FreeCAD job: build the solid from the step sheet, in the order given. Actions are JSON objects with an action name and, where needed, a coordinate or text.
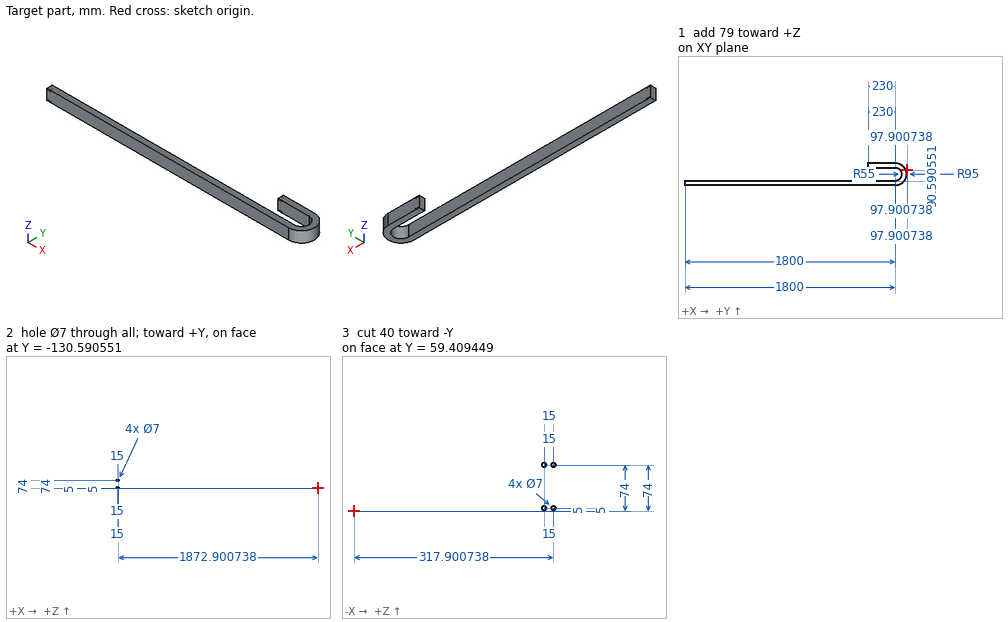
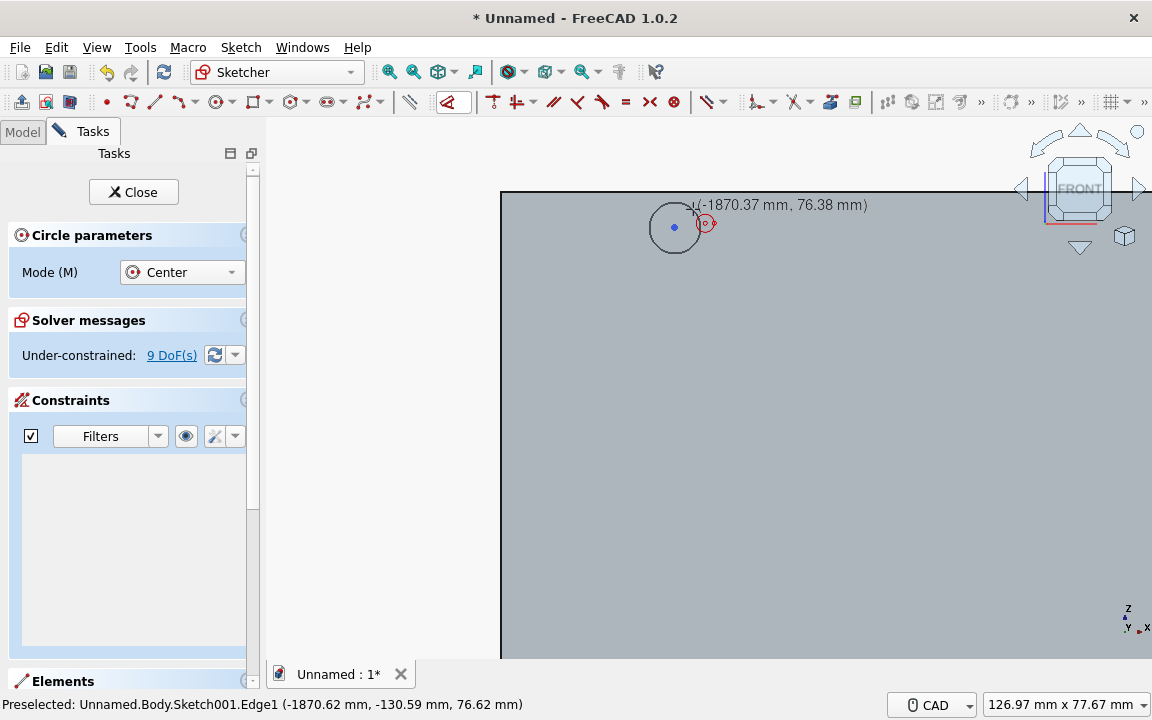
{"action": "left_click", "coordinate": [571, 227]}
{"action": "left_click", "coordinate": [588, 209]}
{"action": "key", "text": "Escape"}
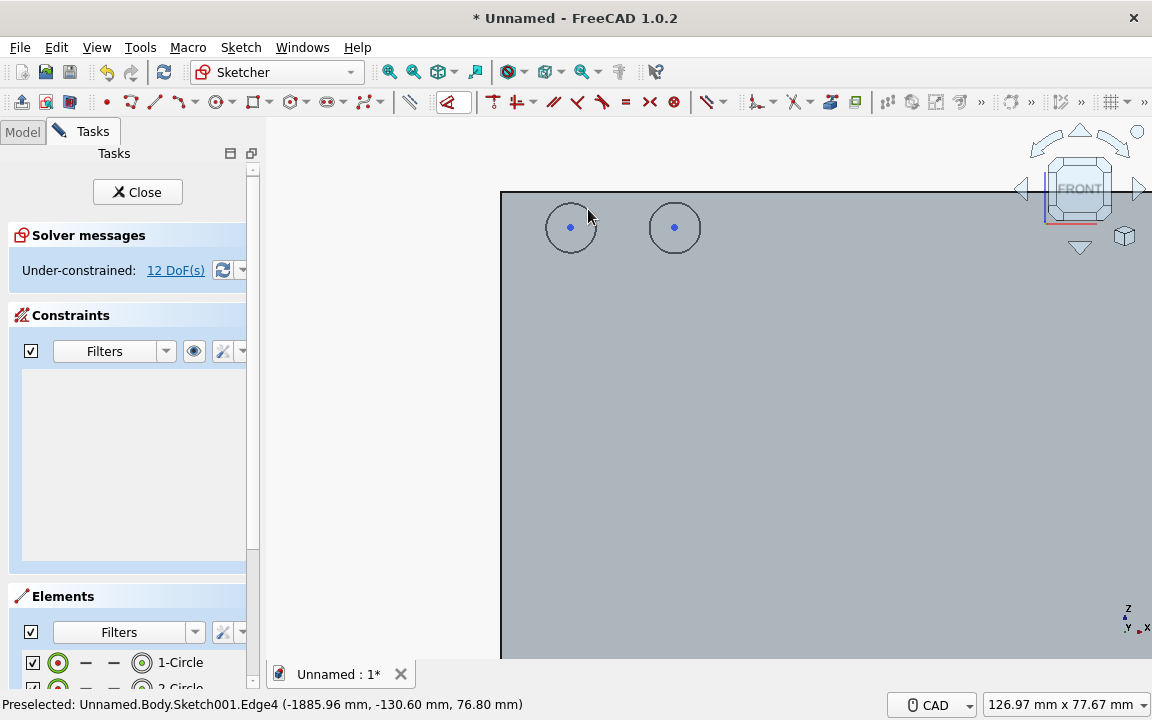
{"action": "scroll", "coordinate": [676, 227], "scroll_direction": "down", "scroll_amount": 2}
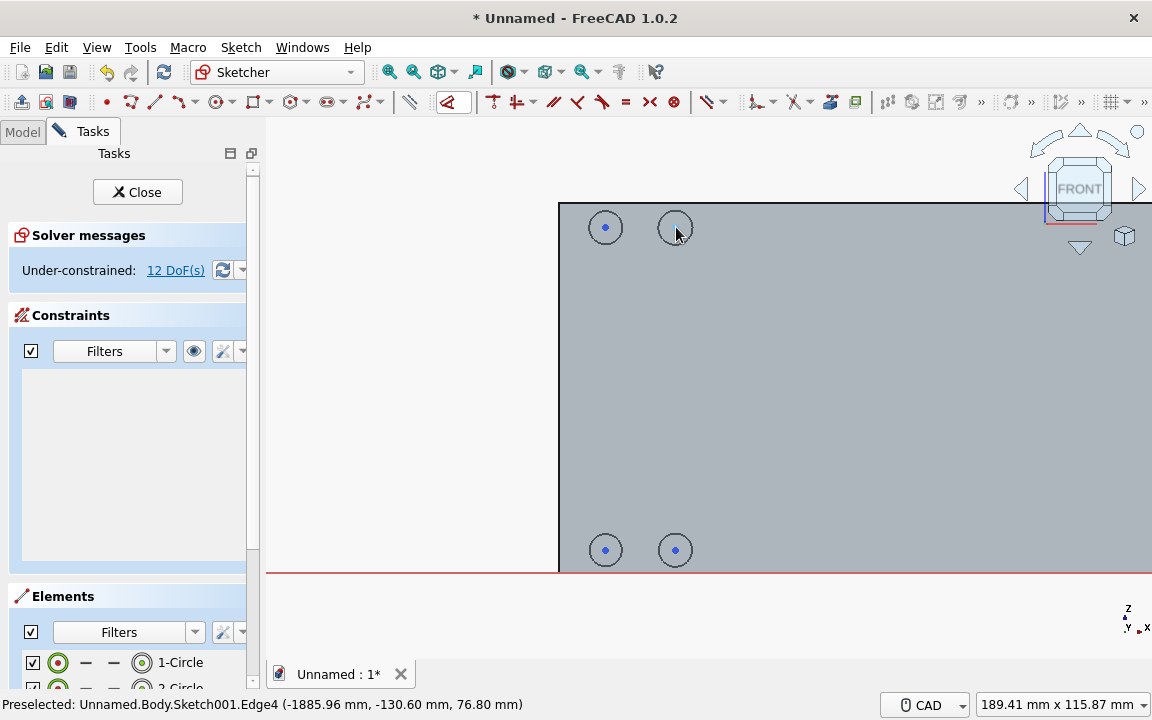
{"action": "left_click", "coordinate": [687, 538]}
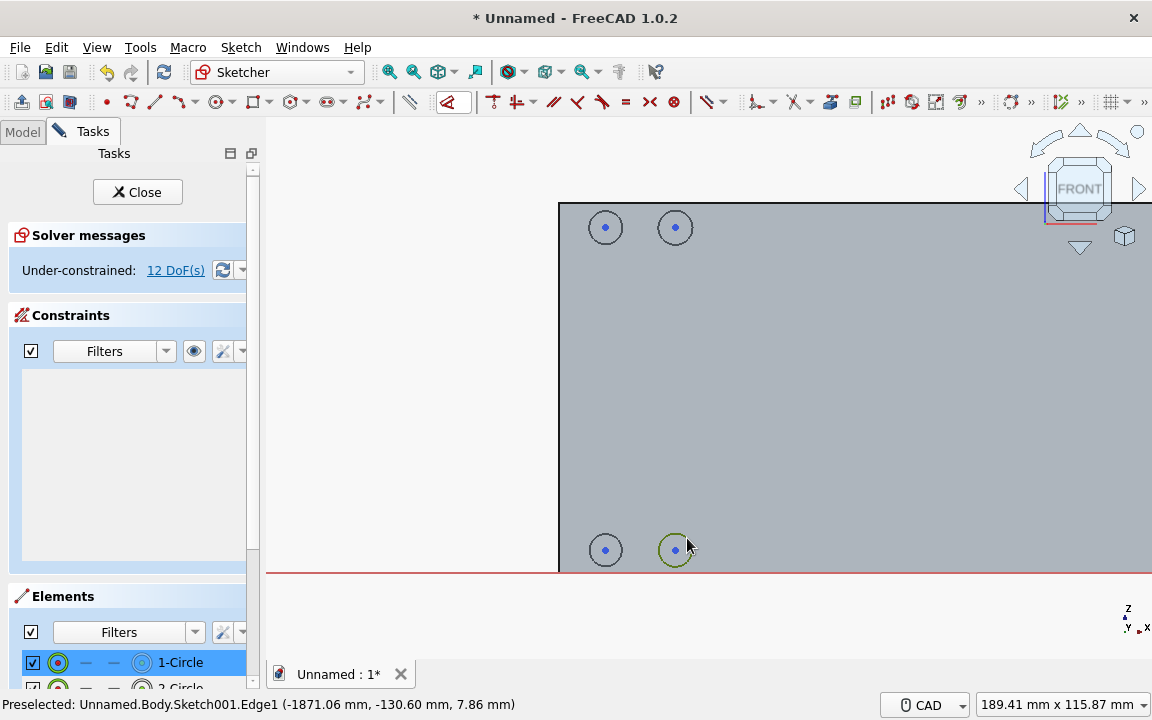
{"action": "left_click", "coordinate": [617, 539]}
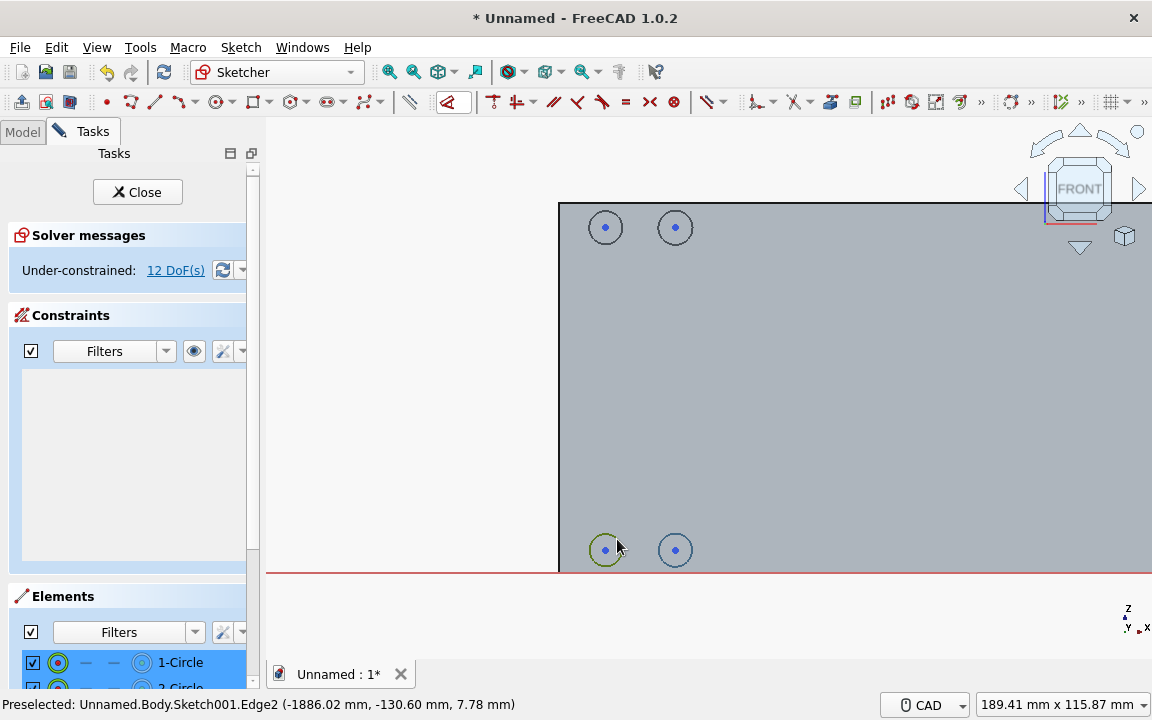
{"action": "left_click", "coordinate": [688, 216]}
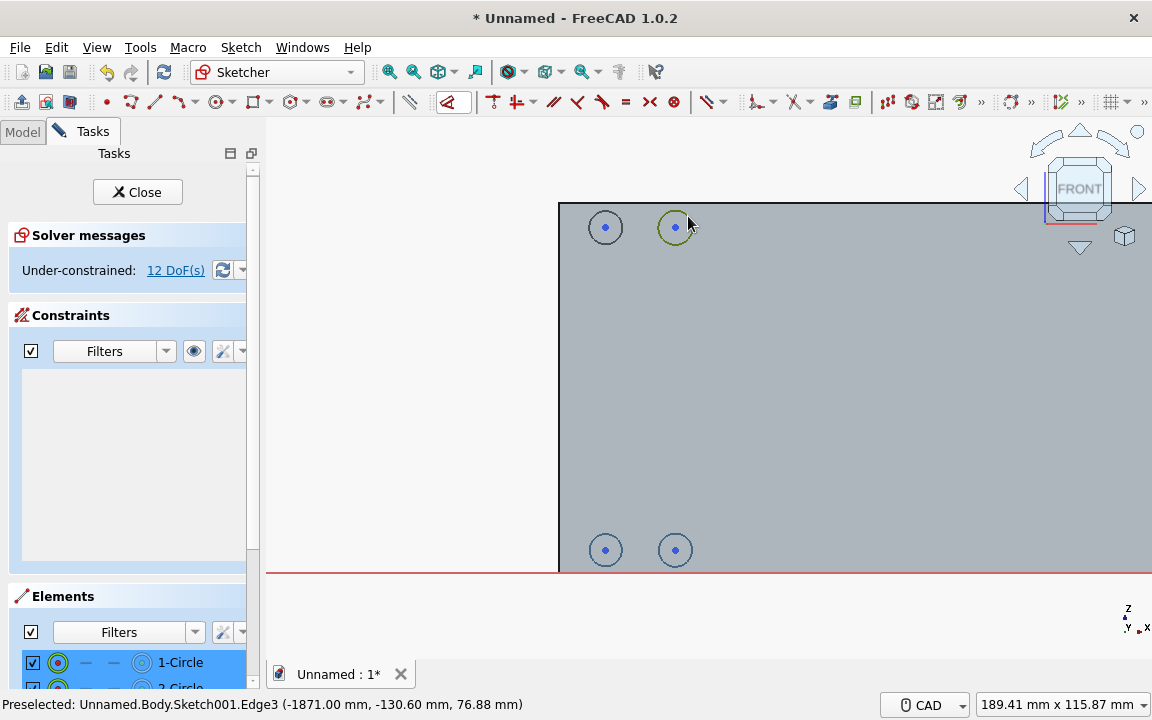
{"action": "left_click", "coordinate": [617, 216]}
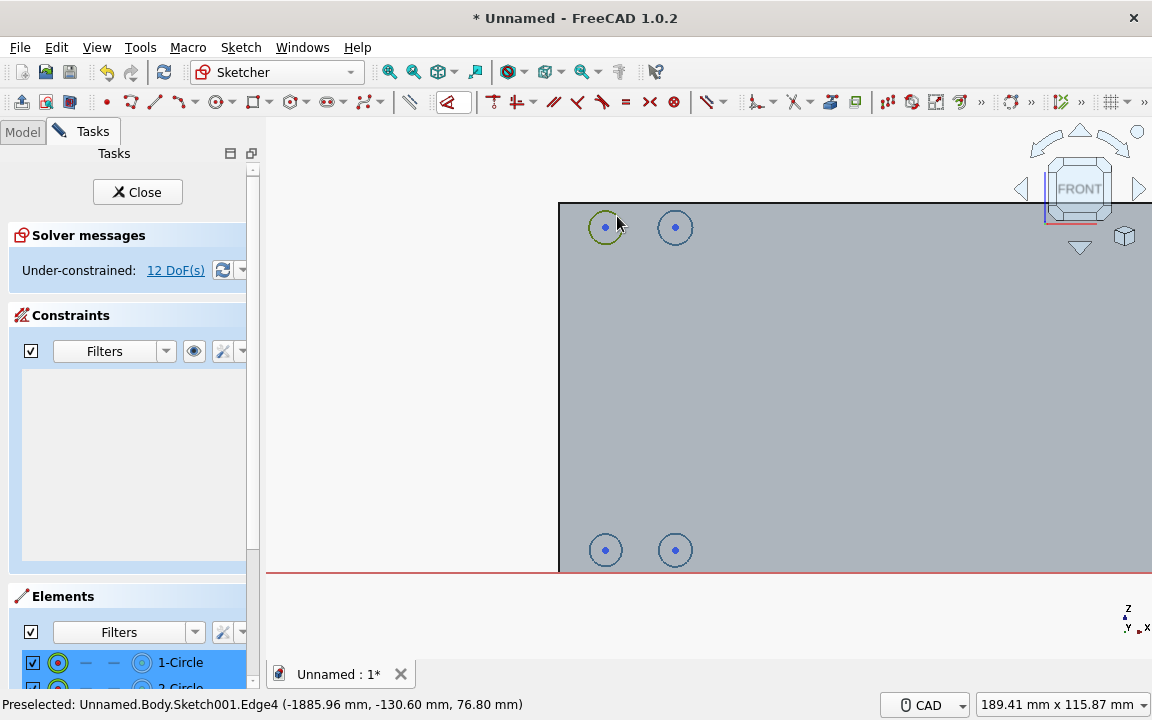
{"action": "left_click", "coordinate": [626, 102]}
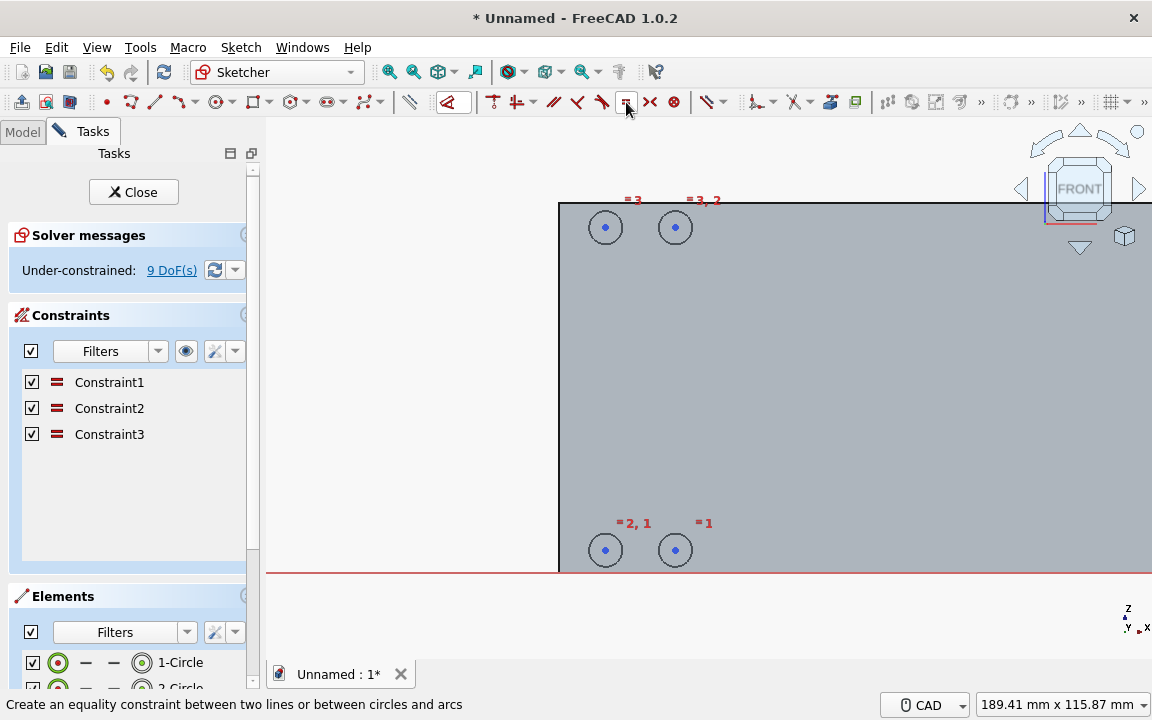
{"action": "key", "text": "d"}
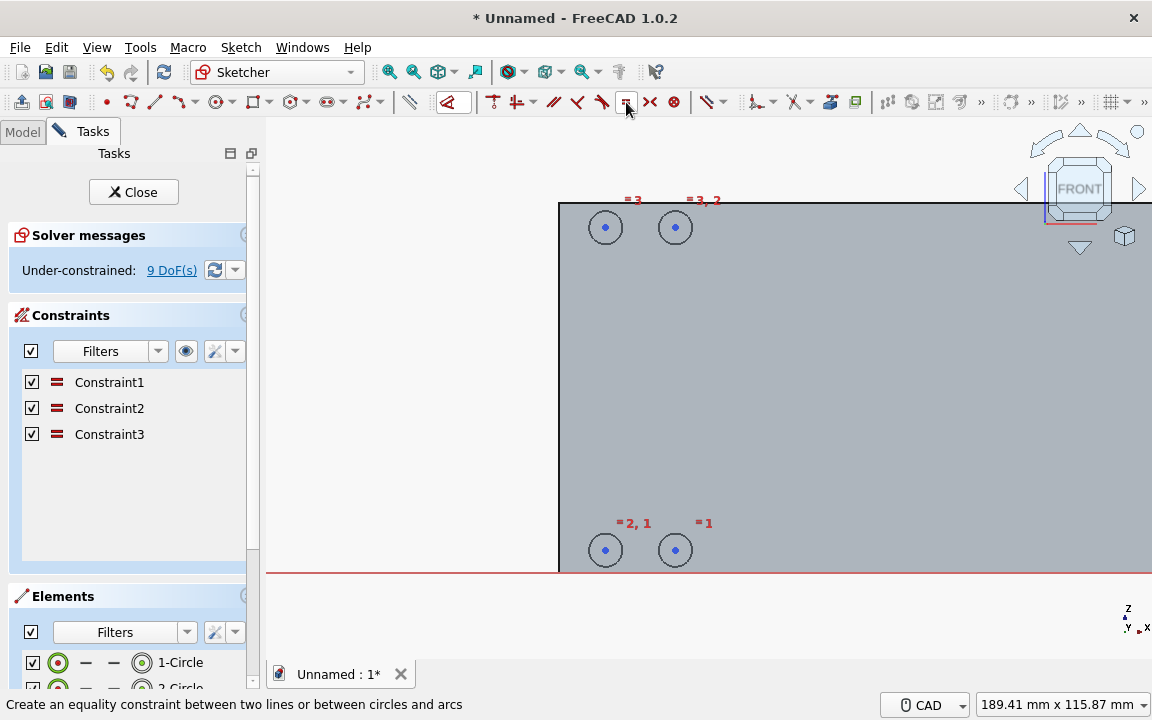
{"action": "left_click", "coordinate": [687, 538]}
{"action": "left_click", "coordinate": [709, 515]}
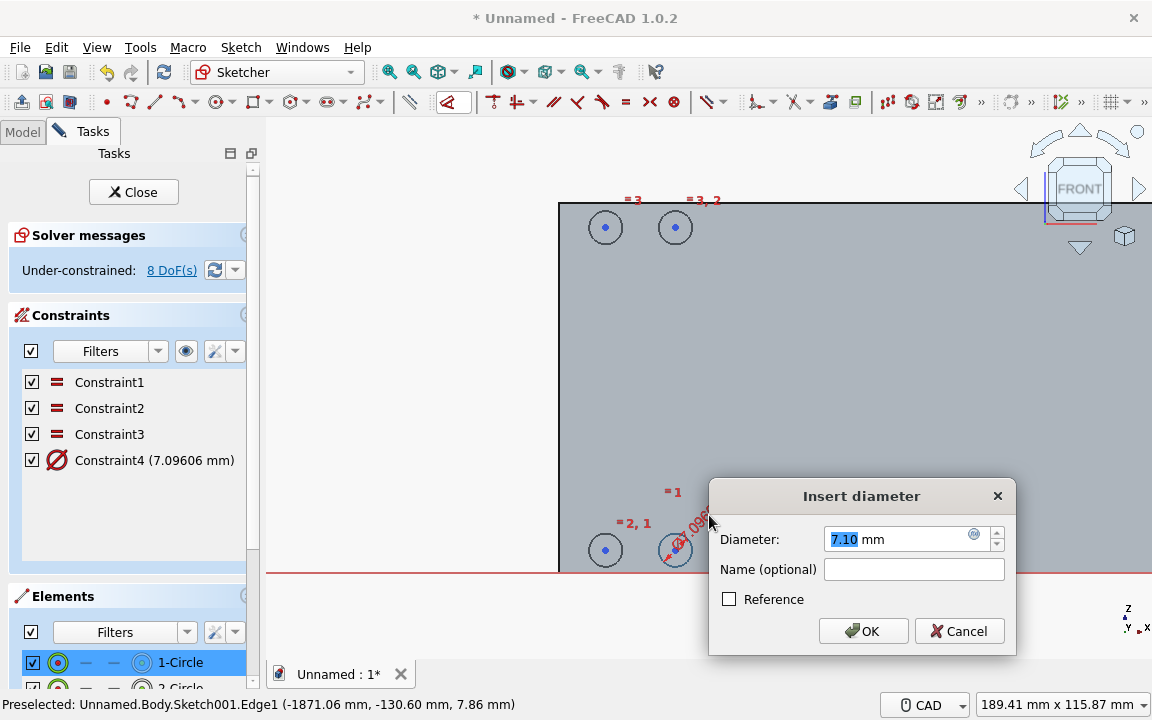
{"action": "type", "text": "7"}
{"action": "key", "text": "Return"}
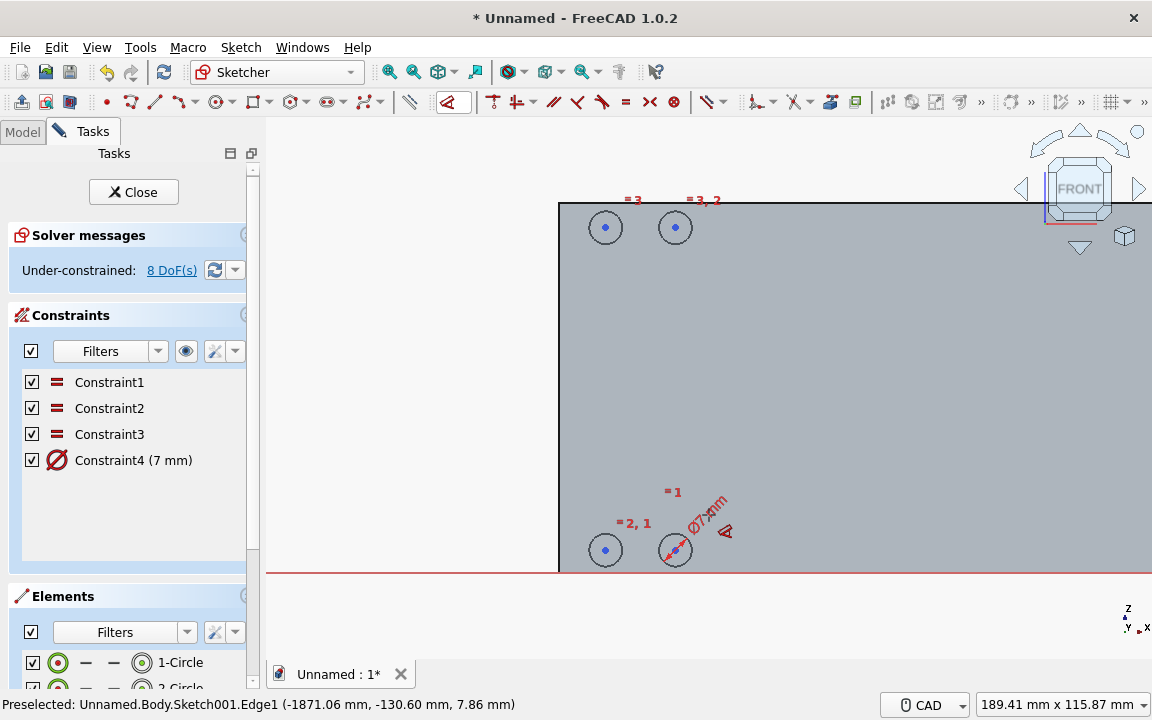
{"action": "scroll", "coordinate": [675, 550], "scroll_direction": "up", "scroll_amount": 3}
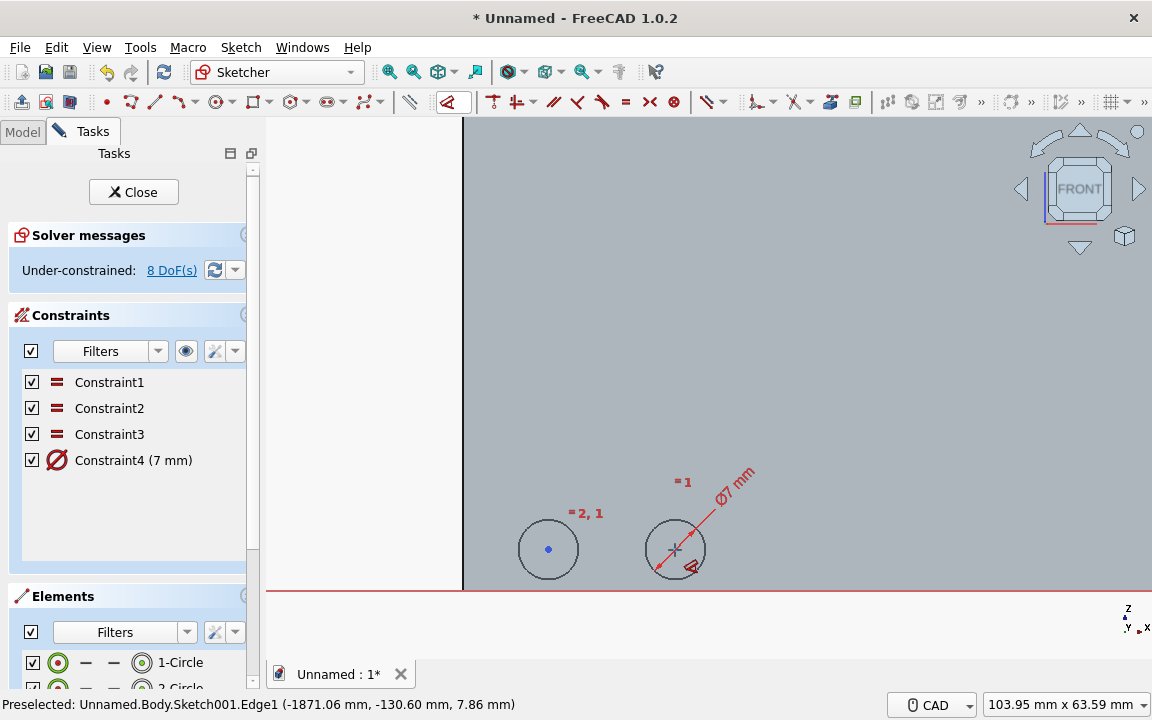
{"action": "left_click", "coordinate": [675, 550]}
{"action": "left_click", "coordinate": [617, 570]}